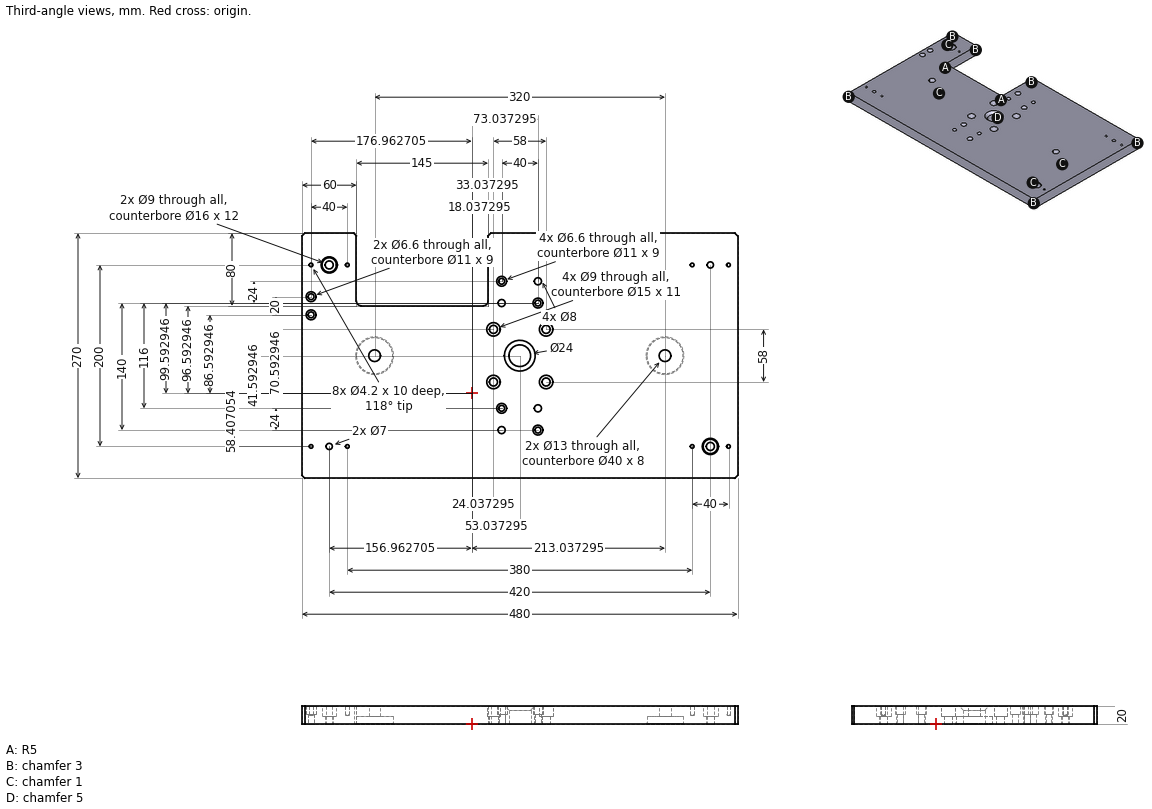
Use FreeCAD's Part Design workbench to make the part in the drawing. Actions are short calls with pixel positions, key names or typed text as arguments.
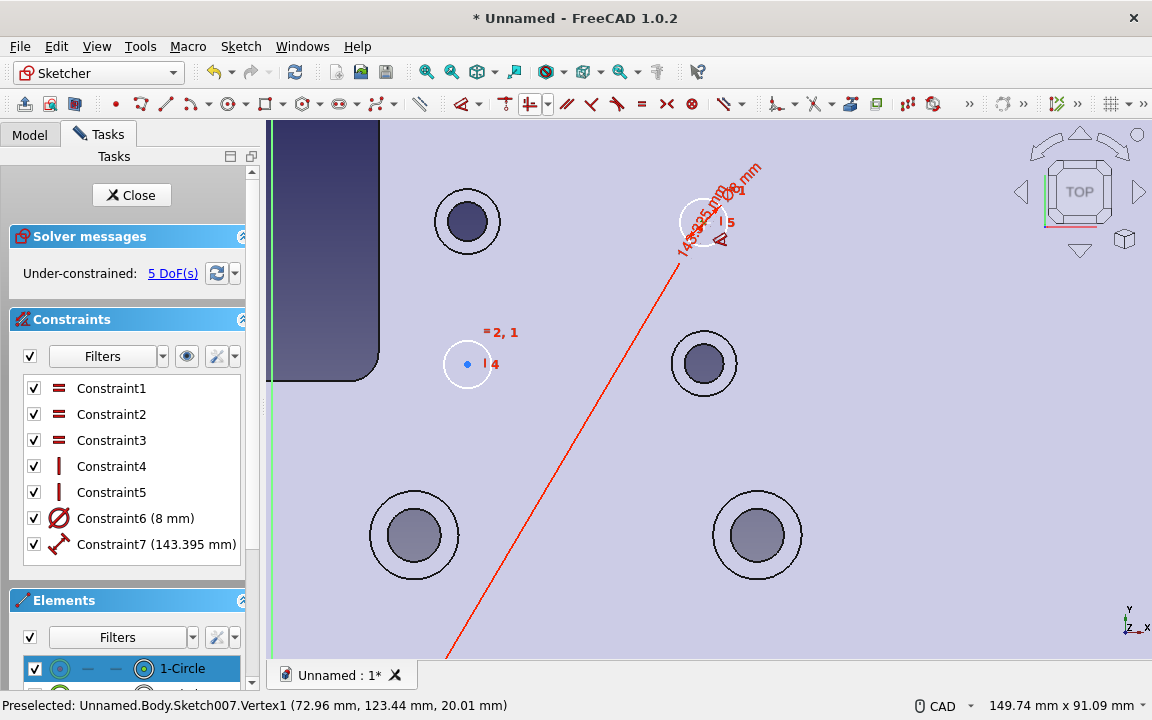
click(468, 365)
click(586, 189)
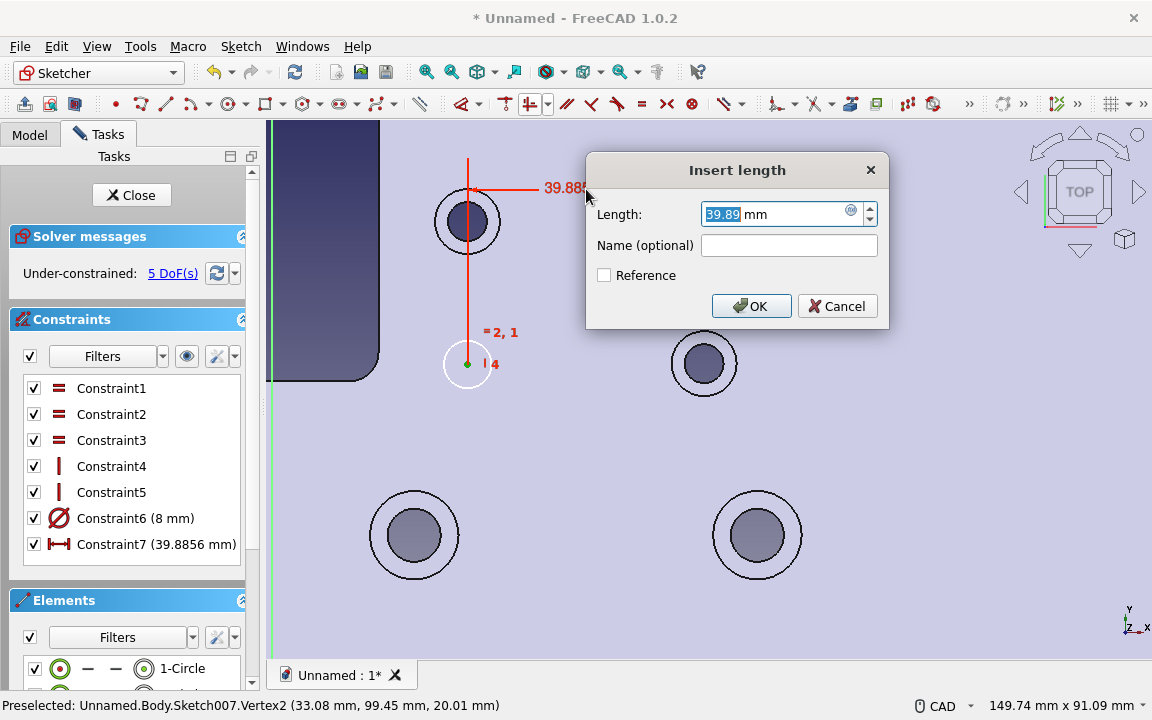
text(40)
key(Return)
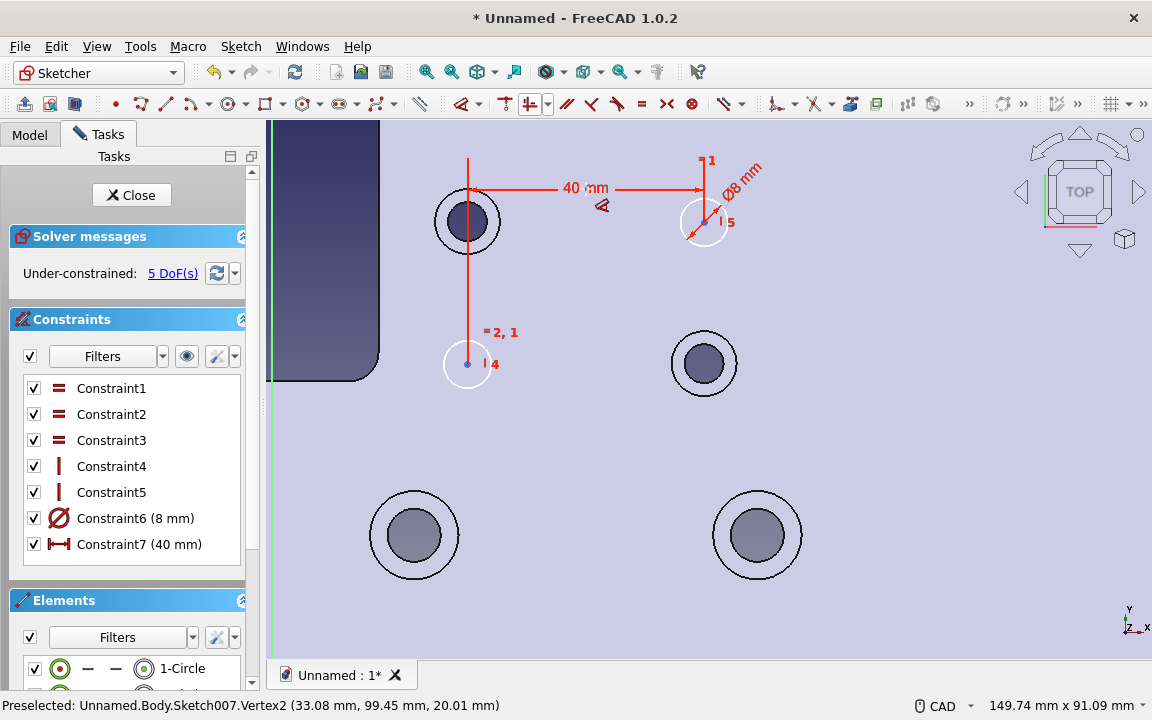
click(704, 223)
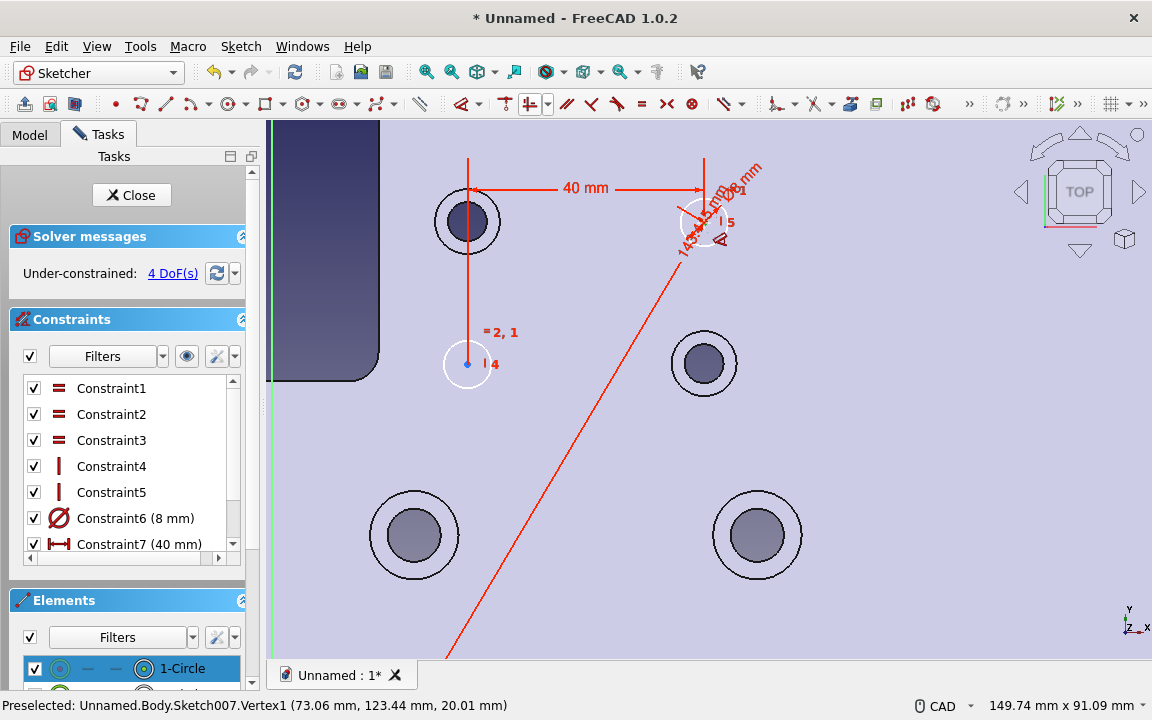
click(468, 365)
click(738, 294)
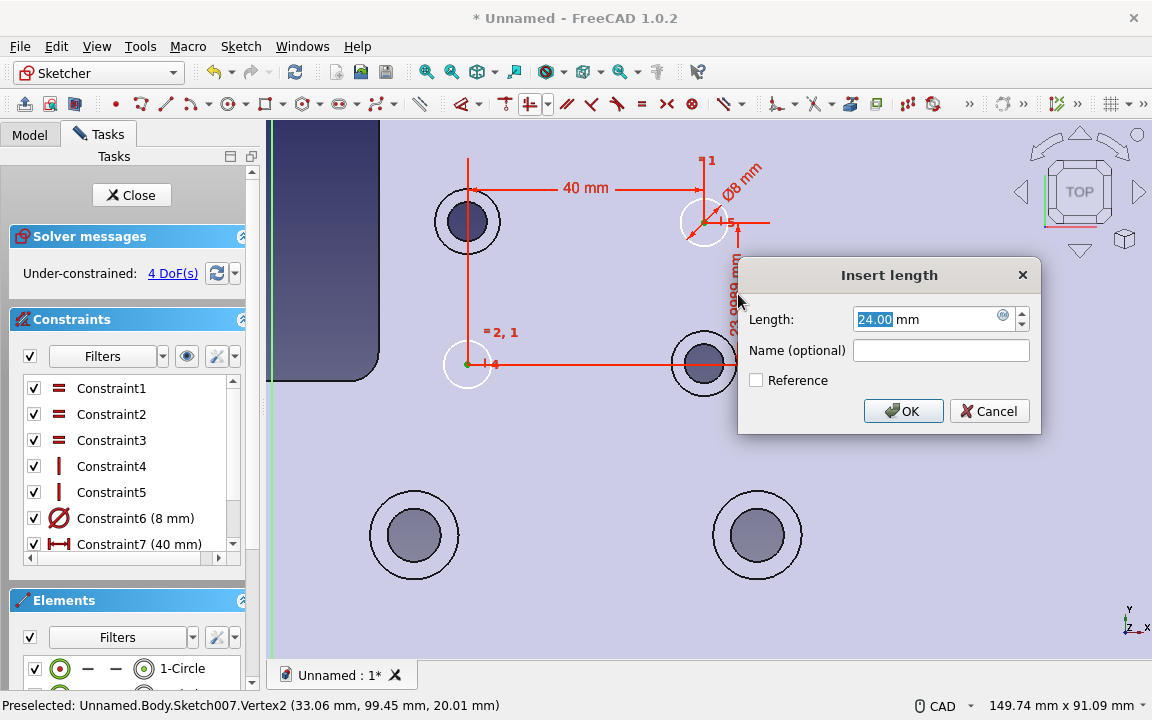
text(24)
key(Return)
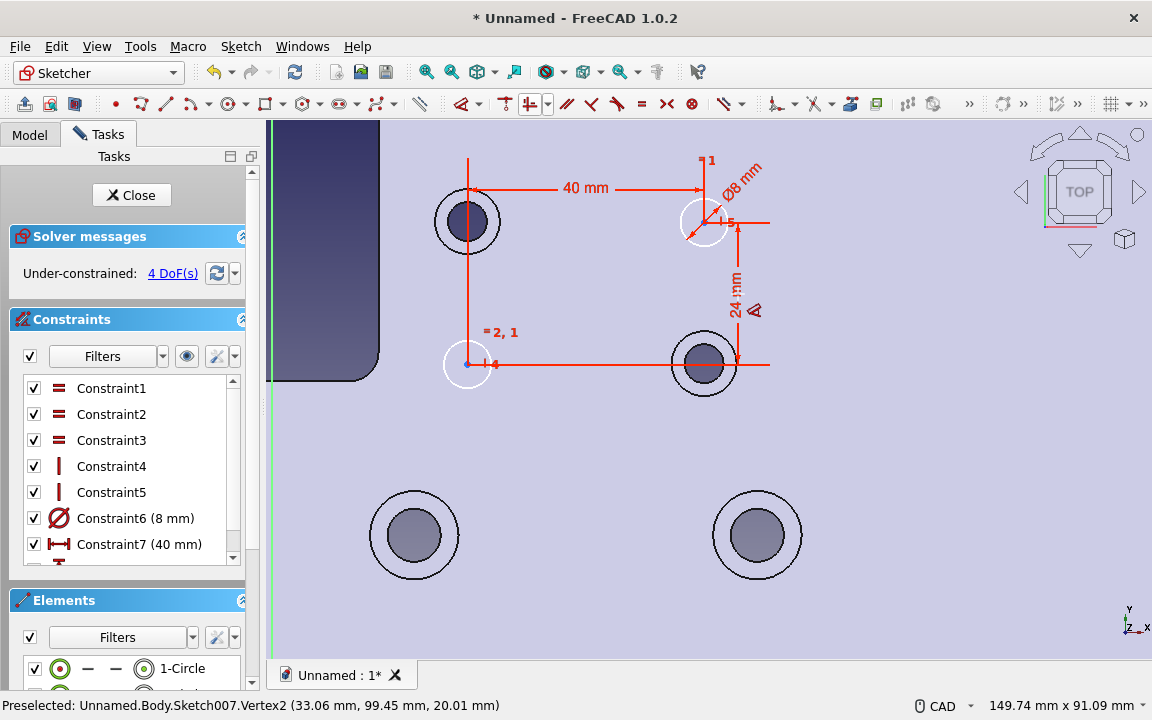
scroll(722, 205, down, 5)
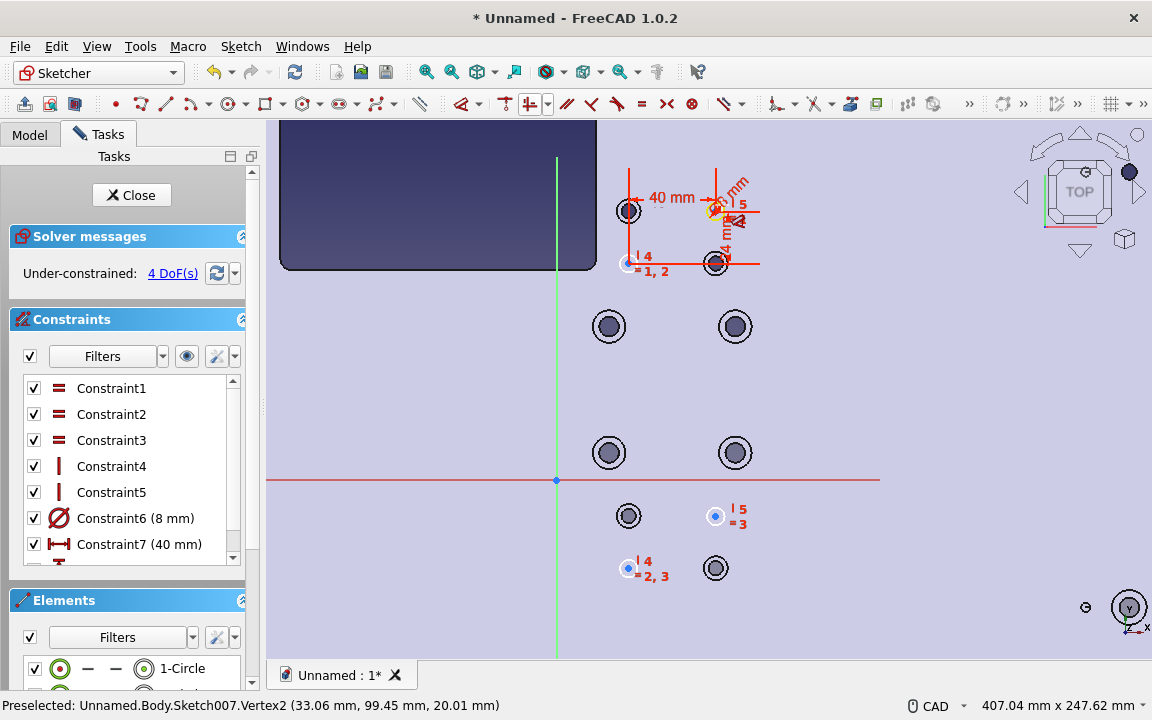
click(629, 569)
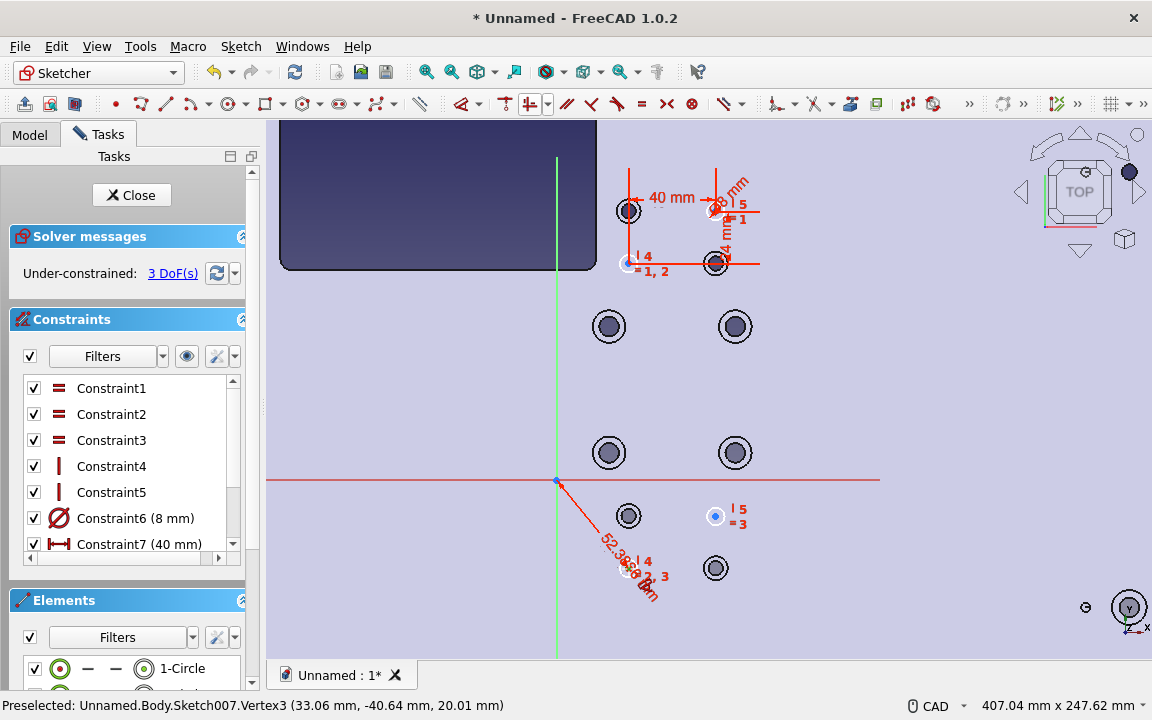
click(716, 516)
click(750, 543)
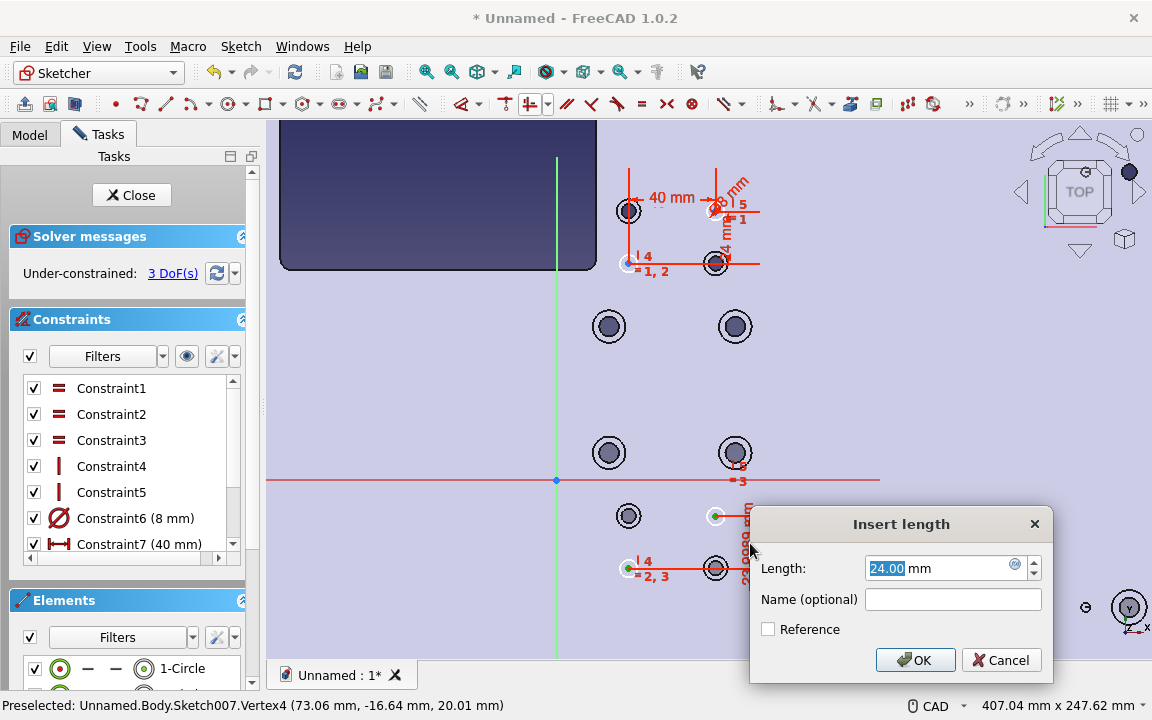
text(24)
key(Return)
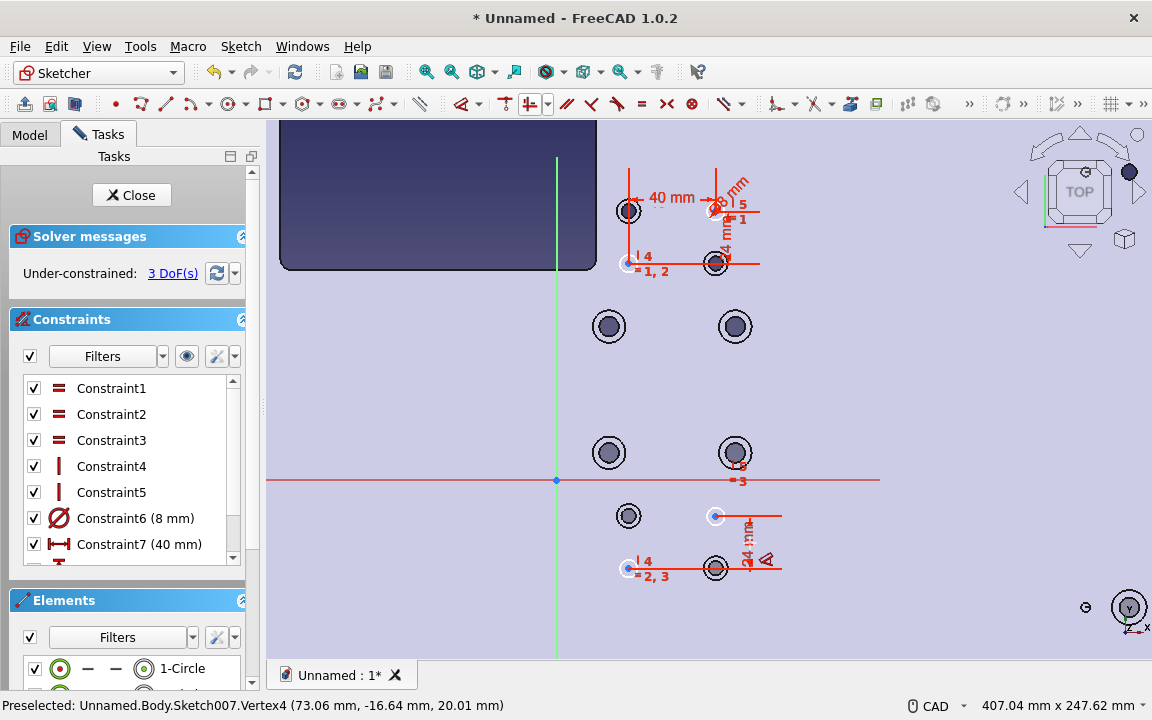
click(629, 264)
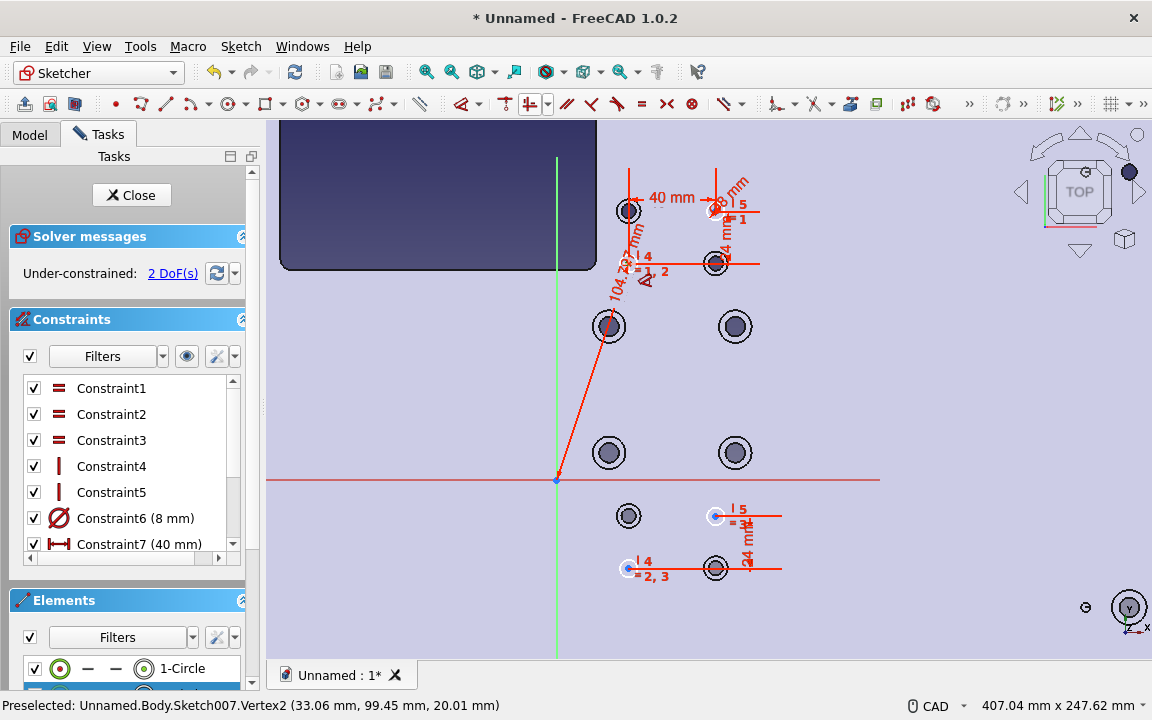
click(629, 569)
click(595, 416)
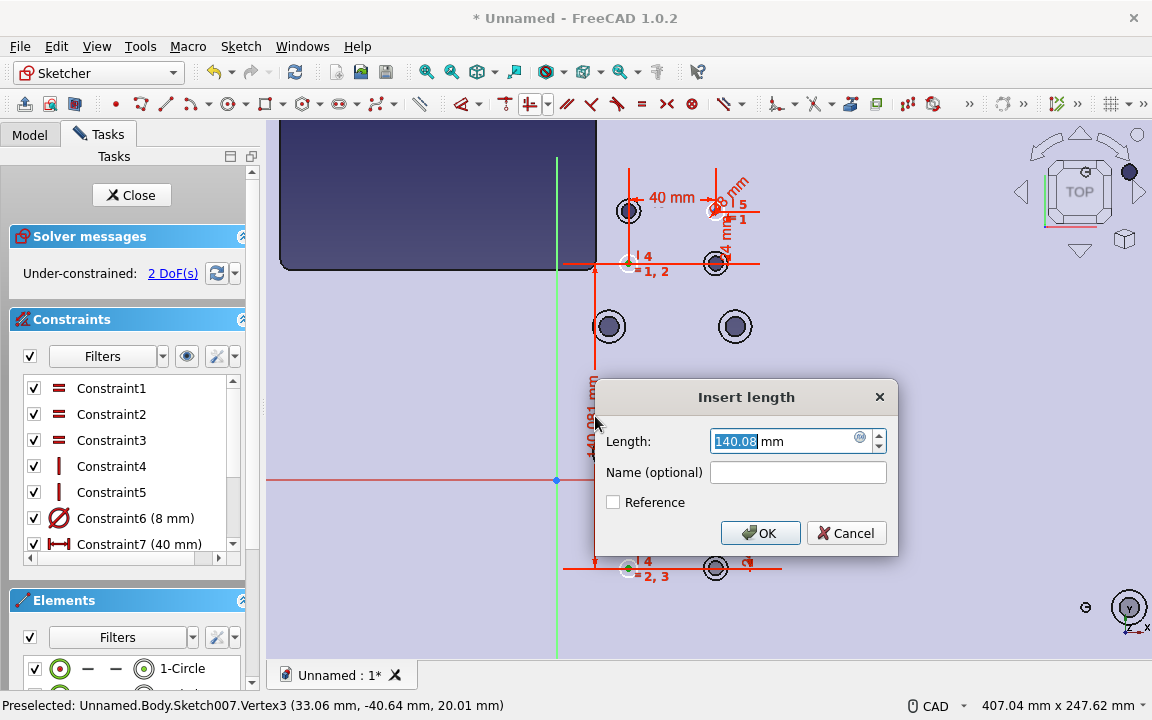
text(140)
key(Return)